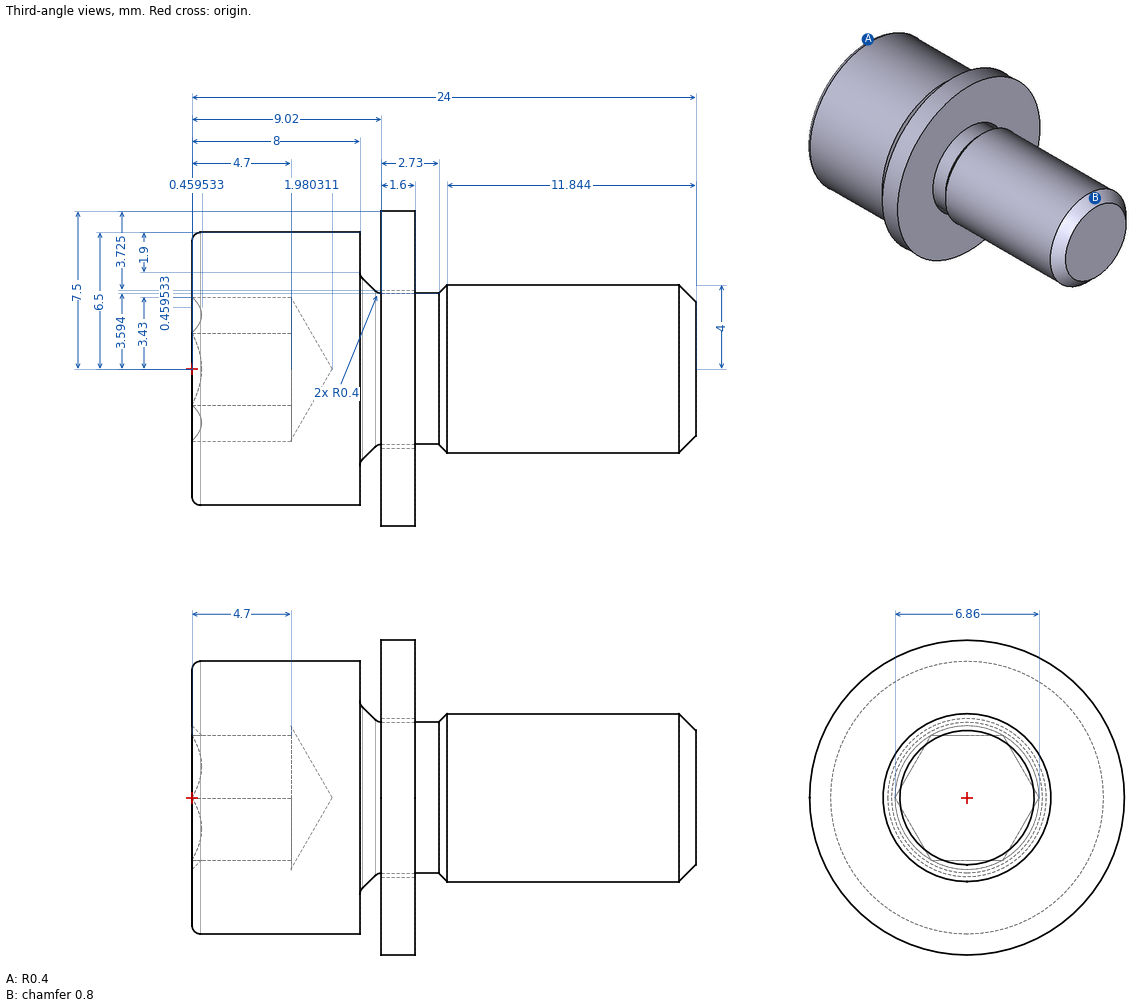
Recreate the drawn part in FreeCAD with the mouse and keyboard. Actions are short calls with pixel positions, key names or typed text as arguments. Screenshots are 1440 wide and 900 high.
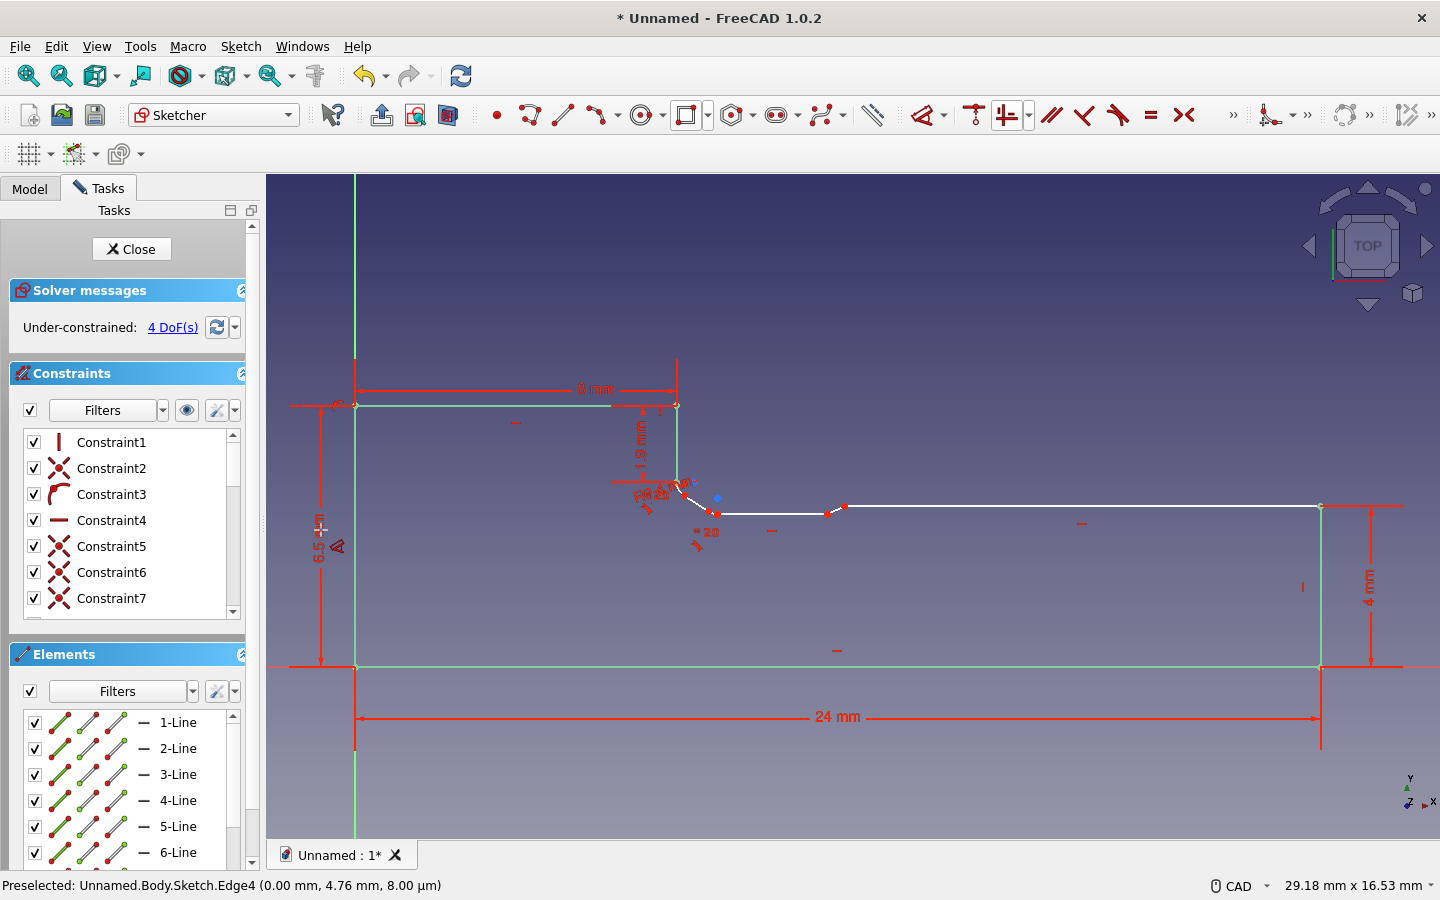
click(795, 514)
click(773, 480)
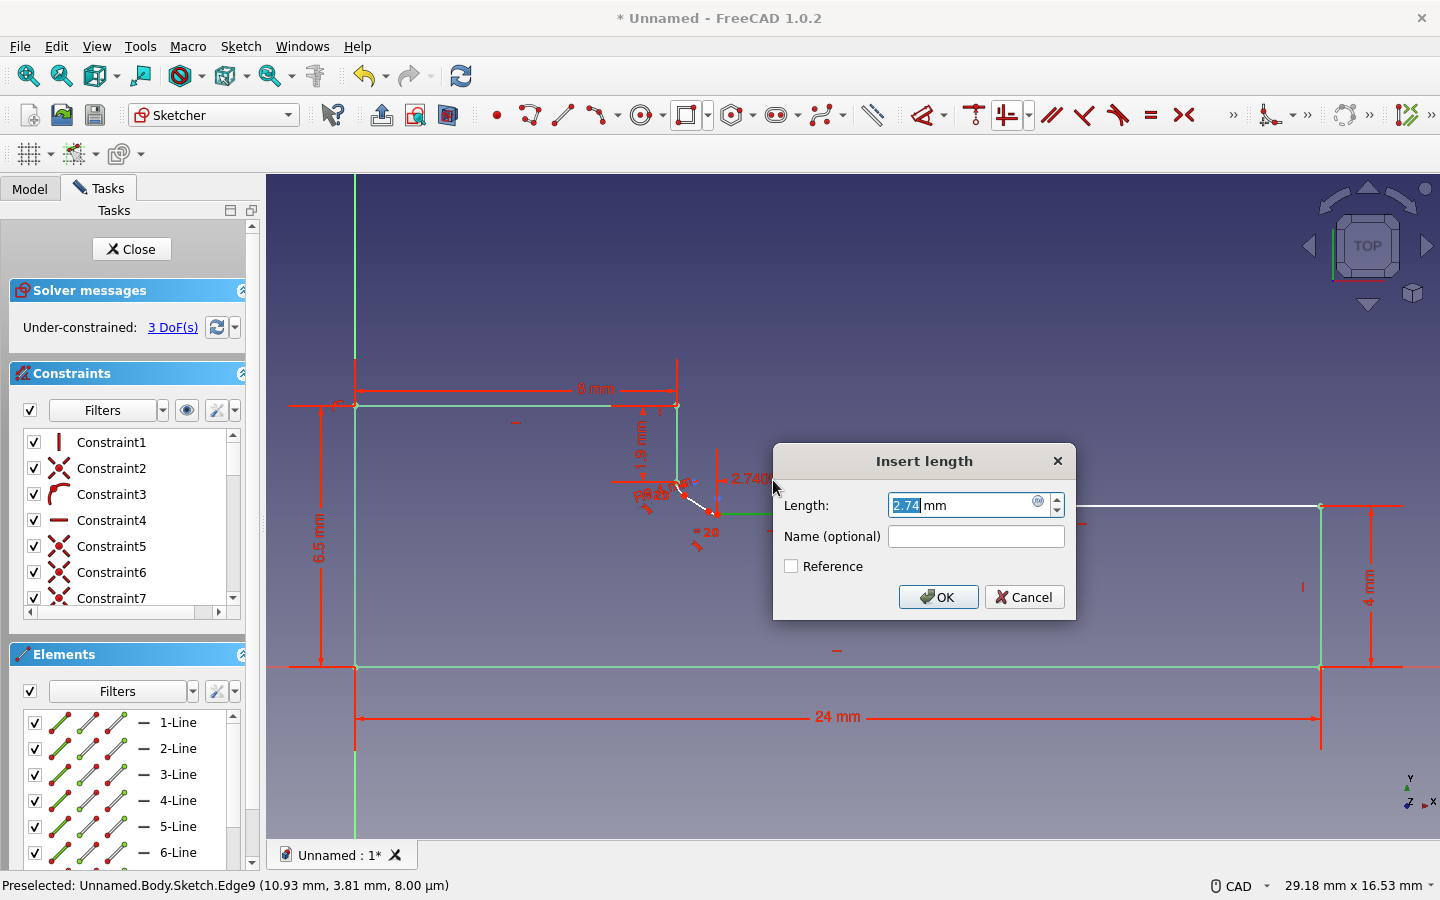
text(2.73)
key(Return)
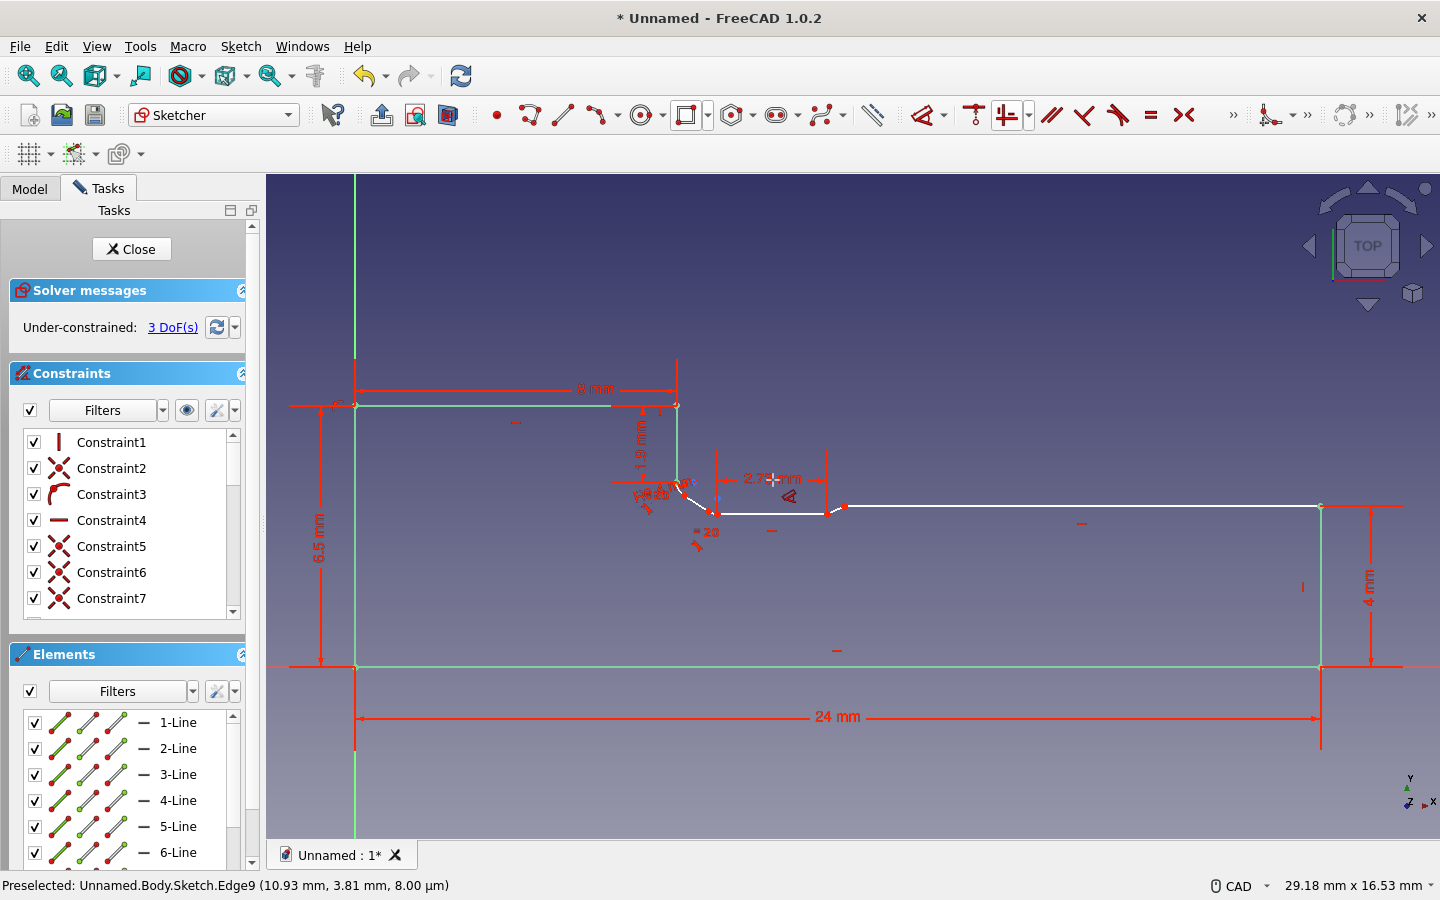
scroll(717, 514, up, 2)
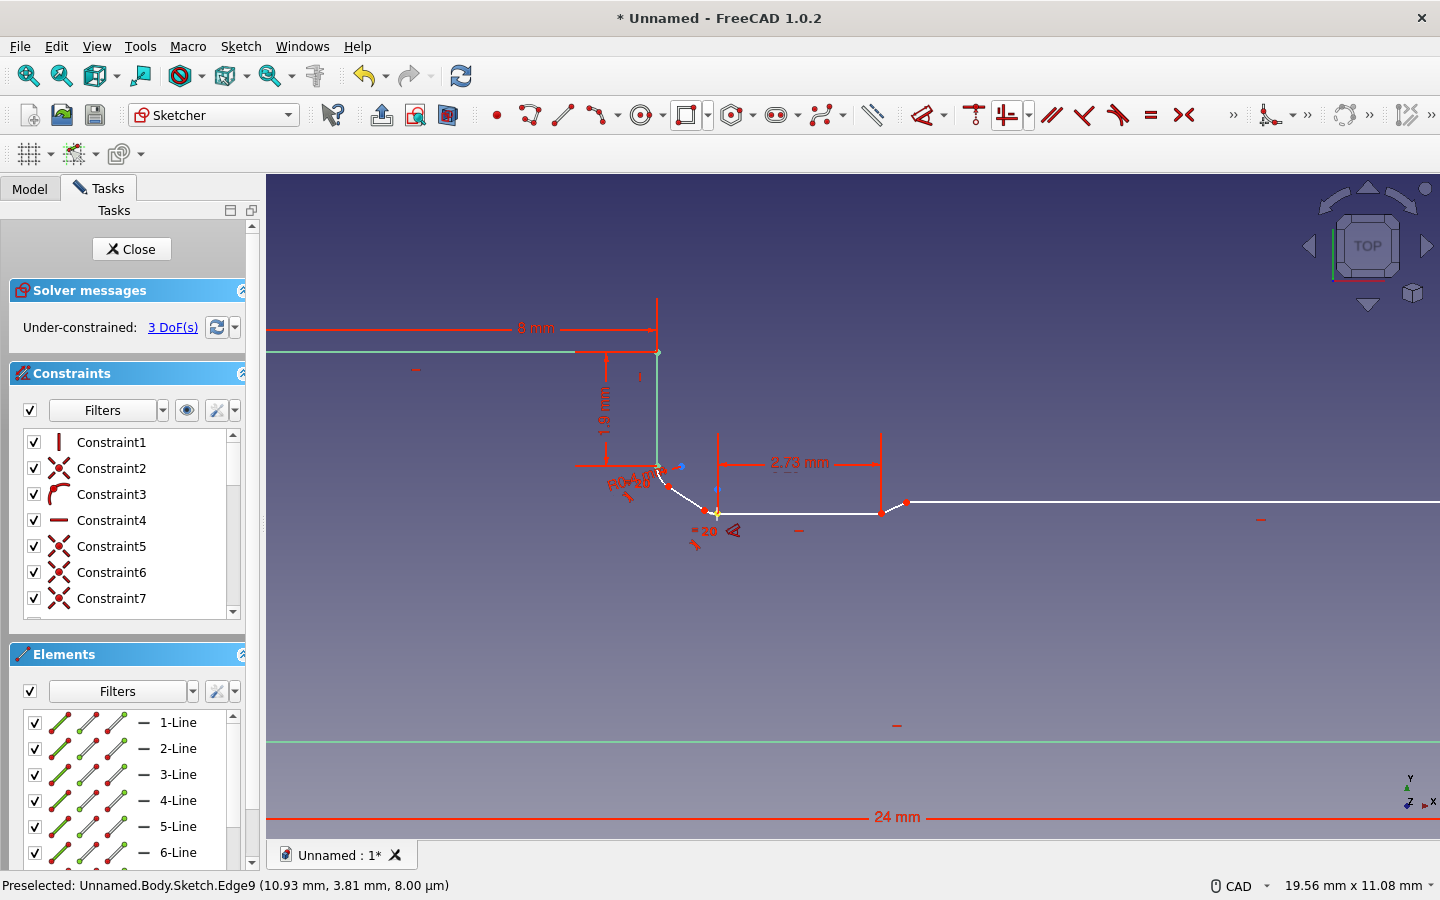
click(718, 514)
click(506, 776)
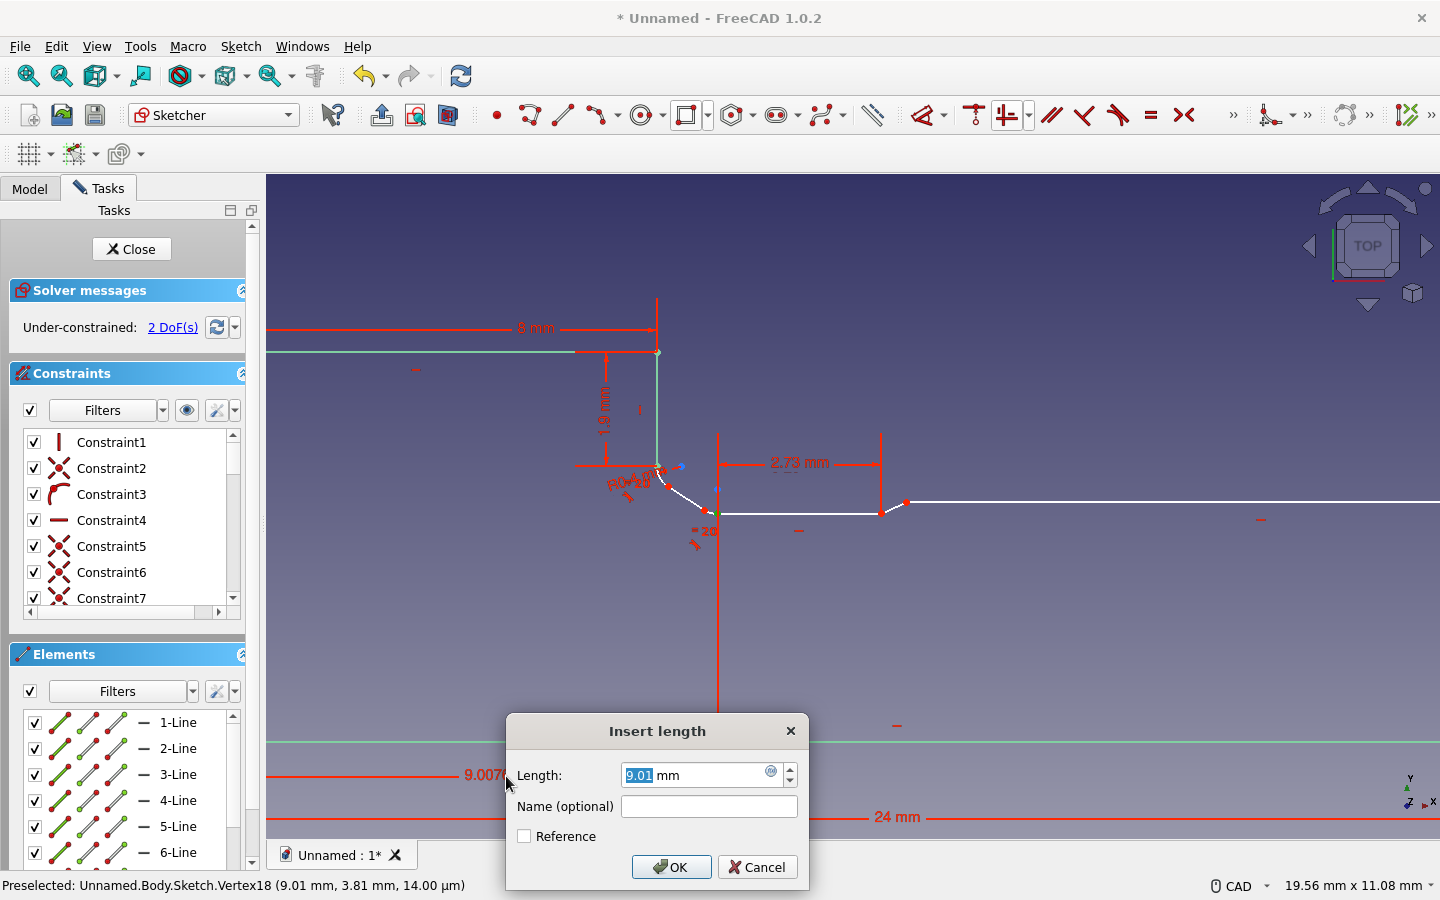
text(9.02)
key(Return)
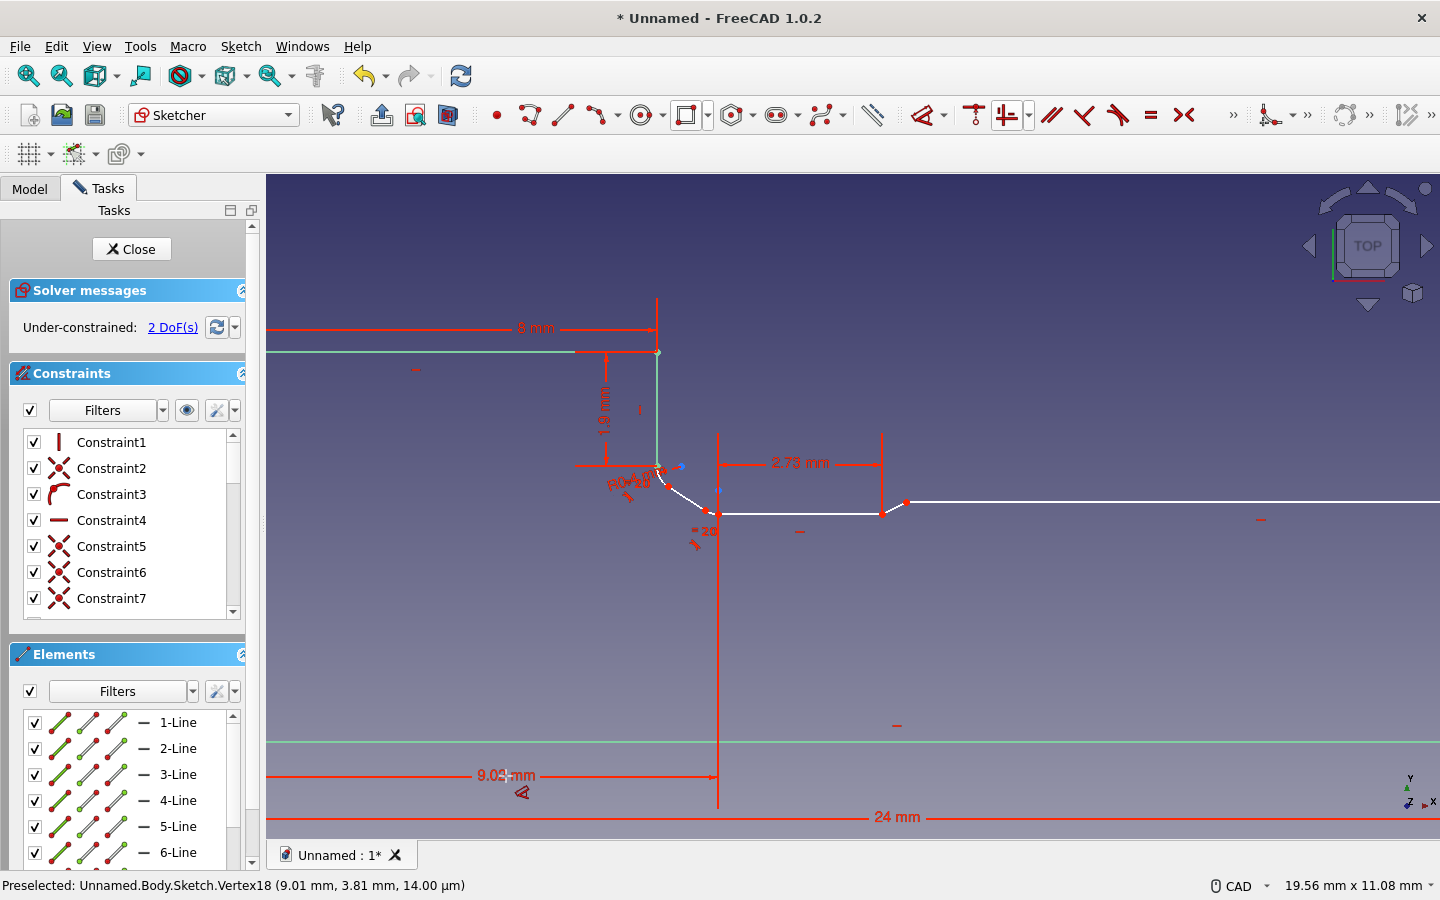
click(1120, 502)
click(1091, 468)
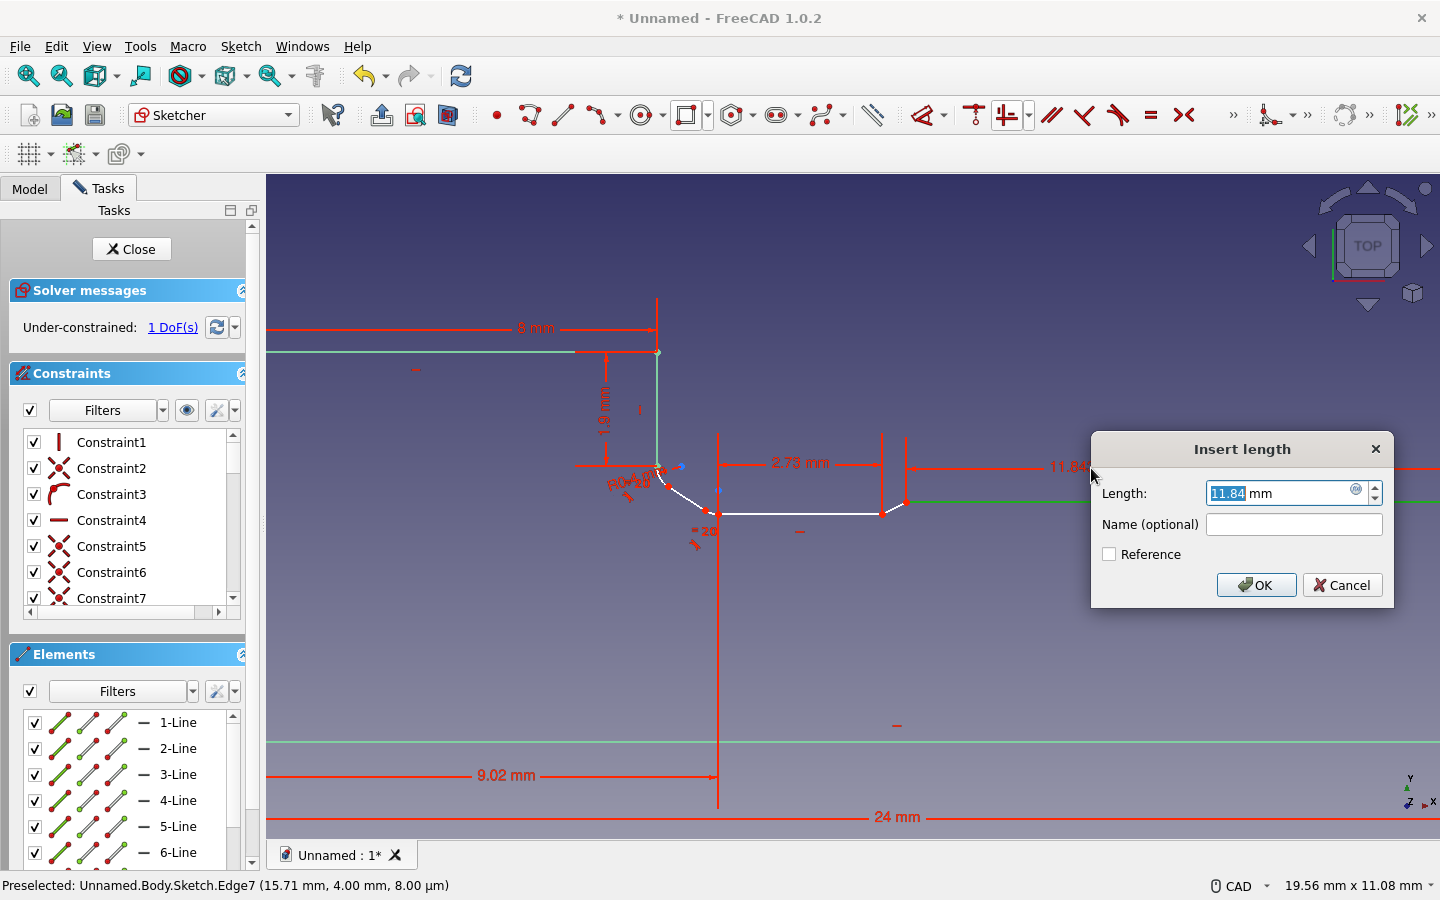
text(11.844)
key(Return)